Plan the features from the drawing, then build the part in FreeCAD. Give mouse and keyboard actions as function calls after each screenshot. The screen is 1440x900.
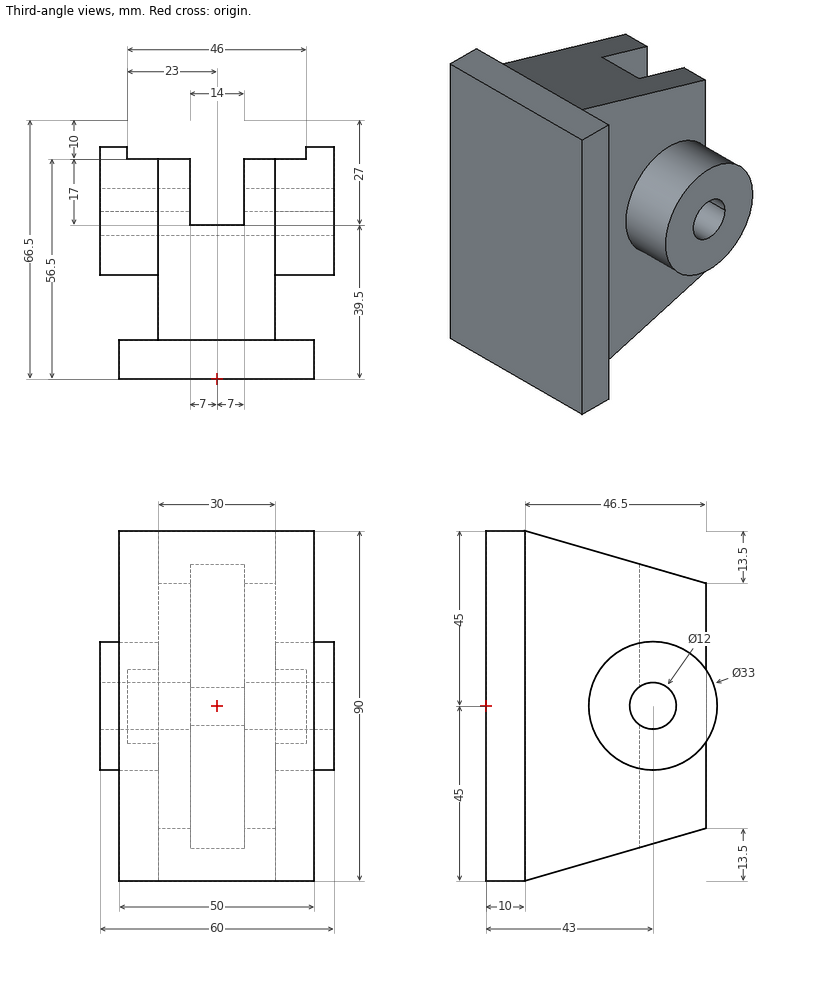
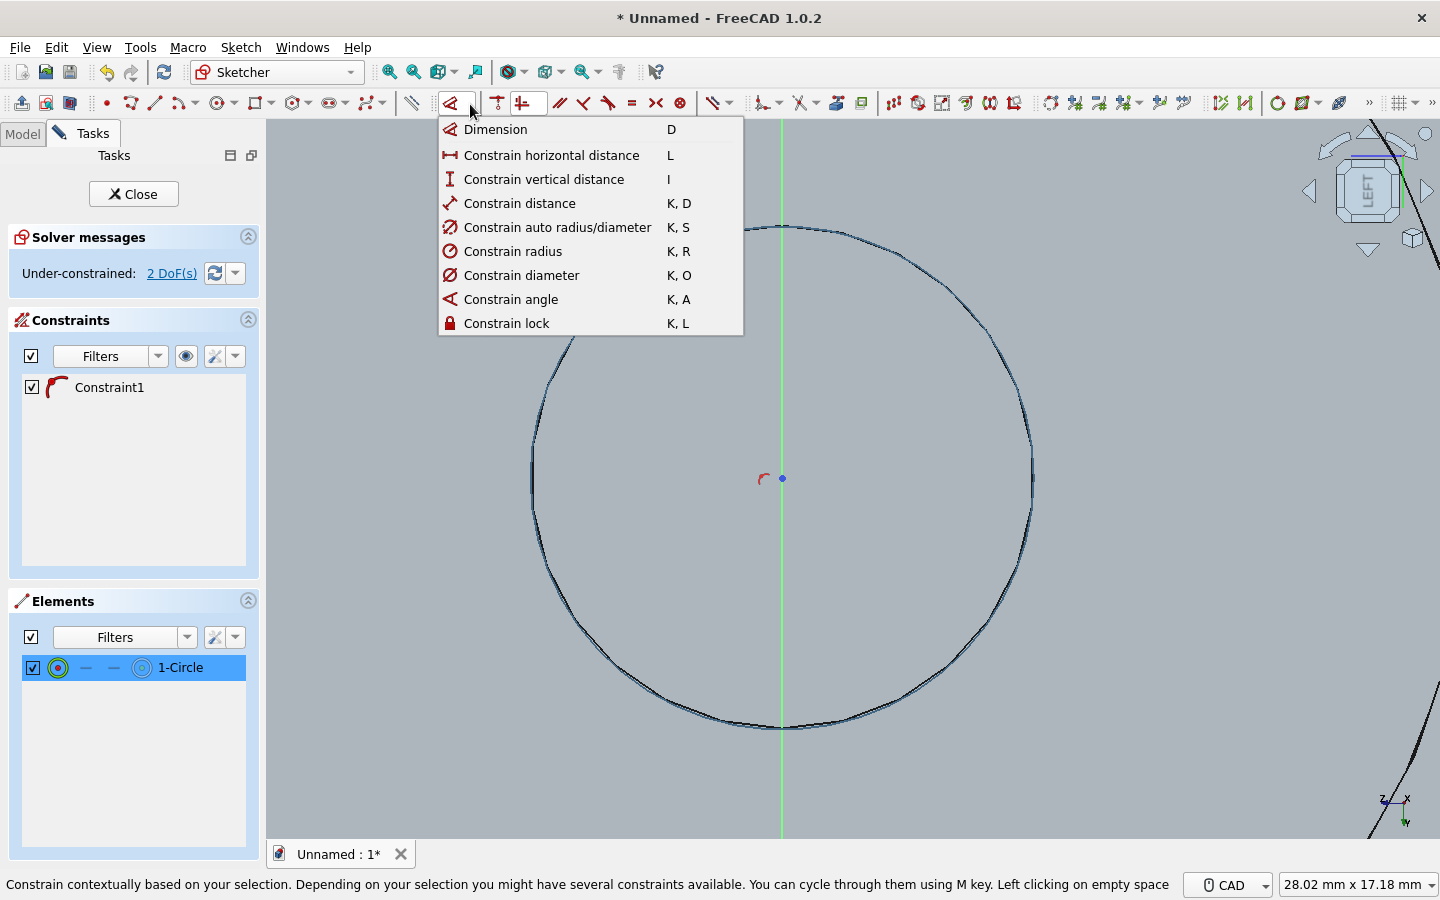
click(591, 275)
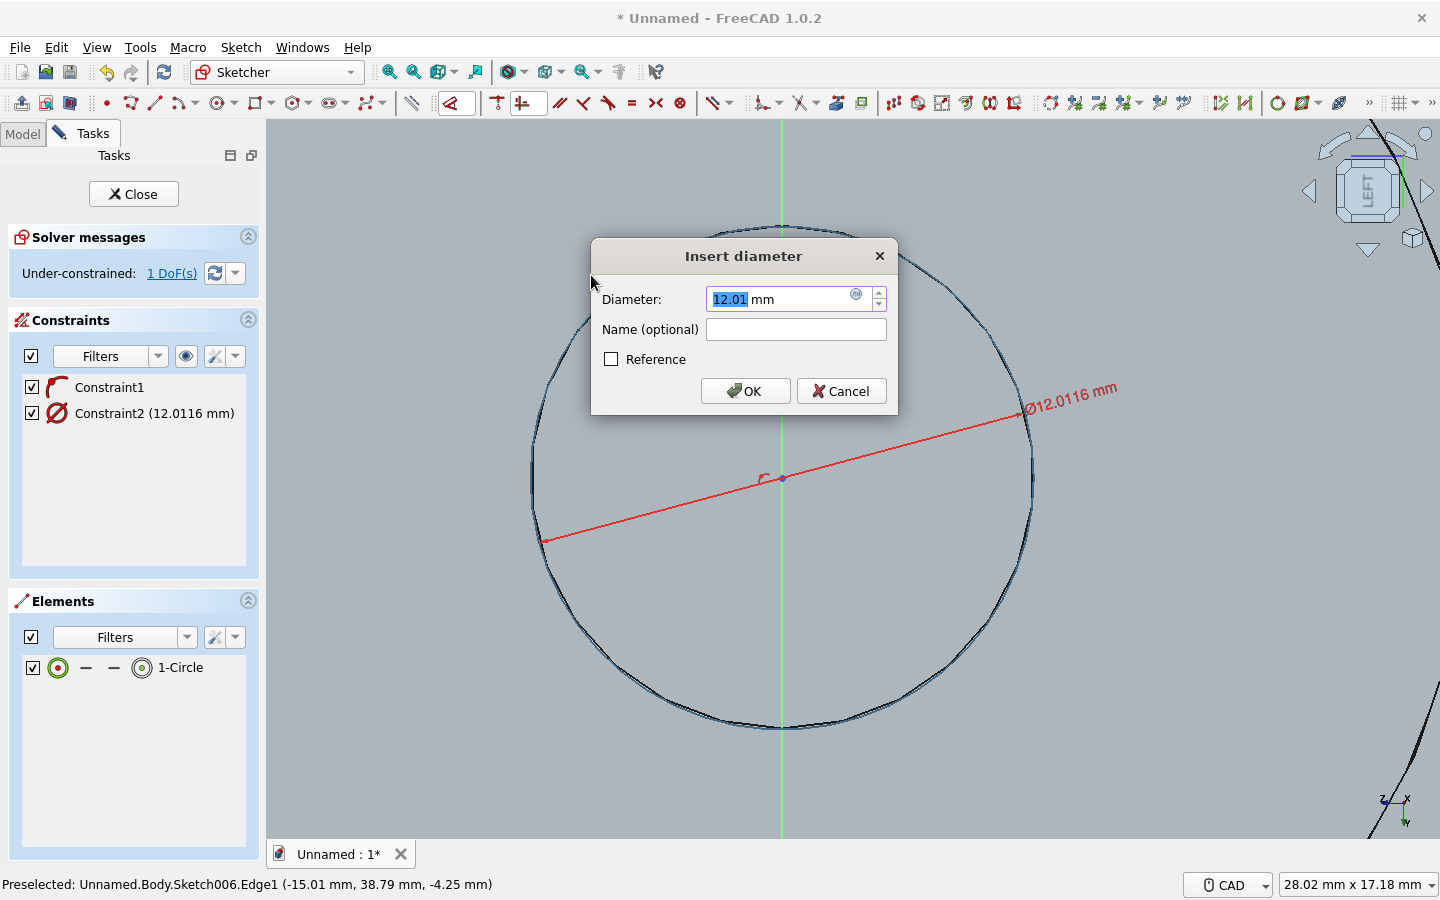
text(12)
key(Return)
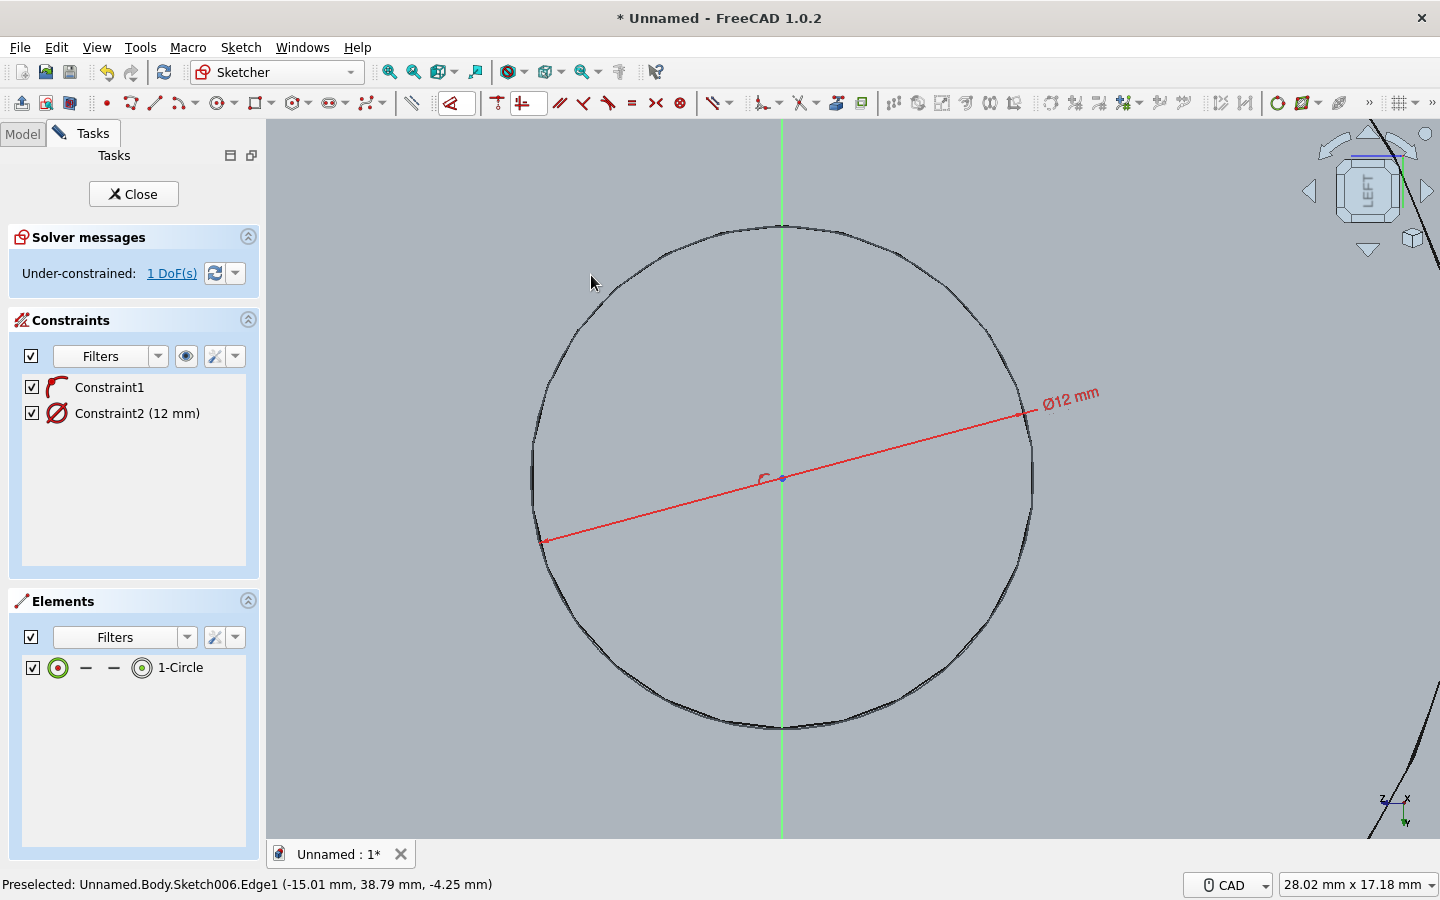
click(782, 478)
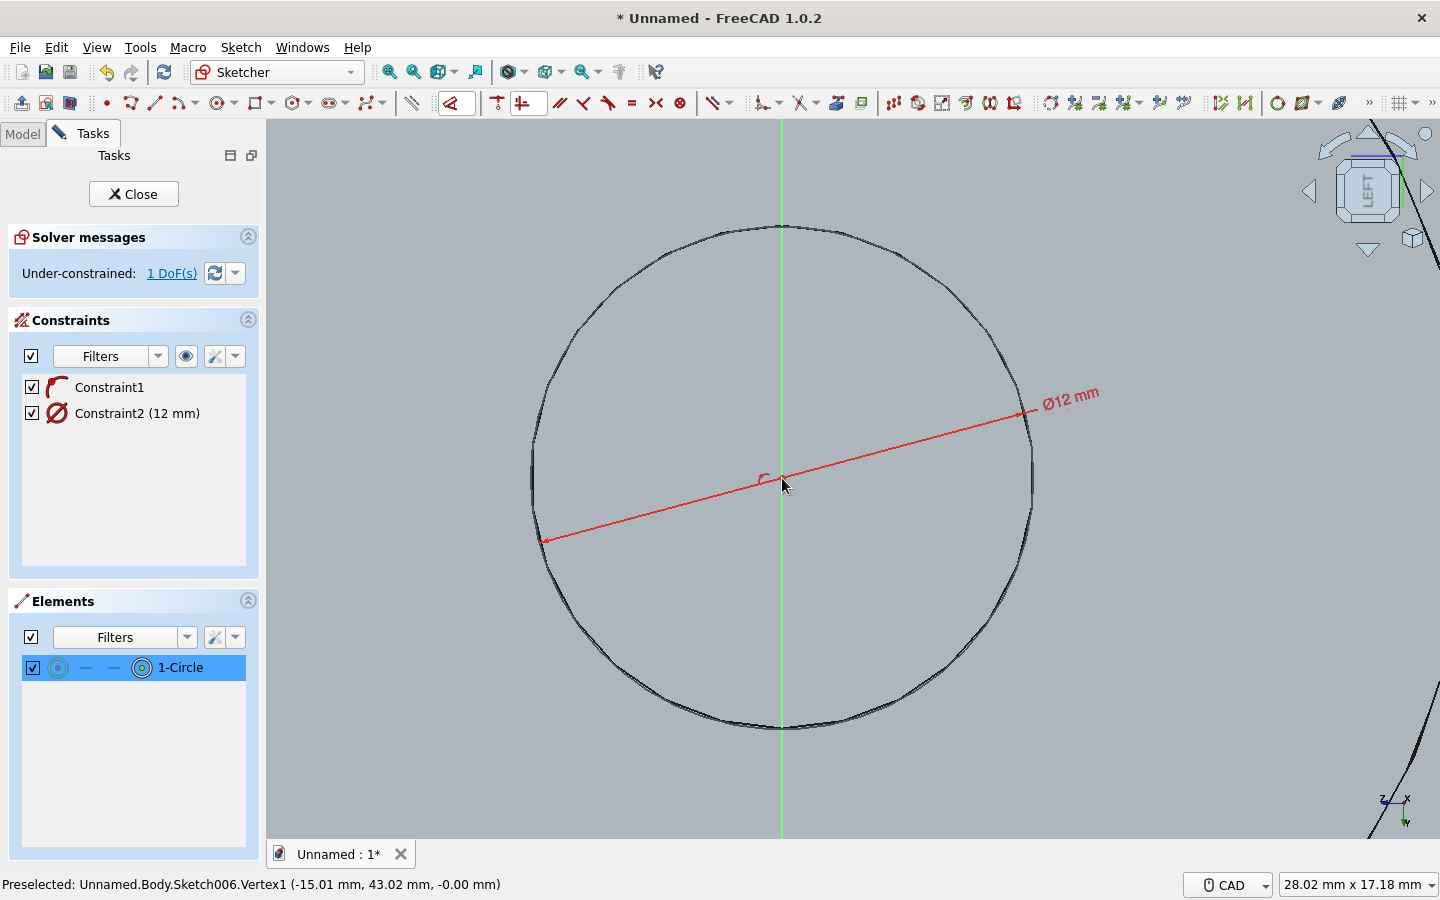
click(470, 104)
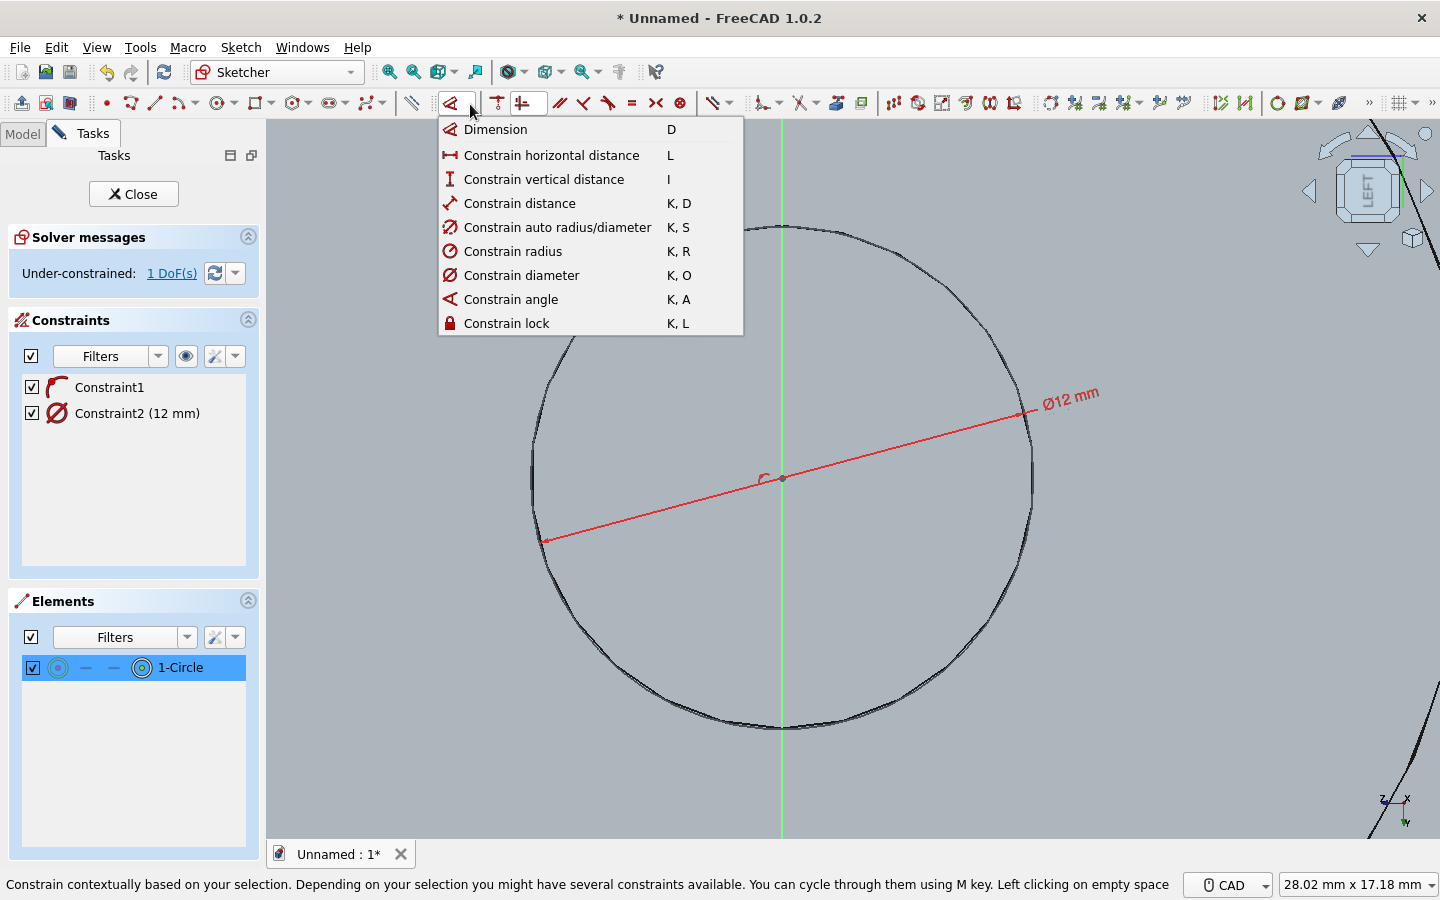
click(591, 179)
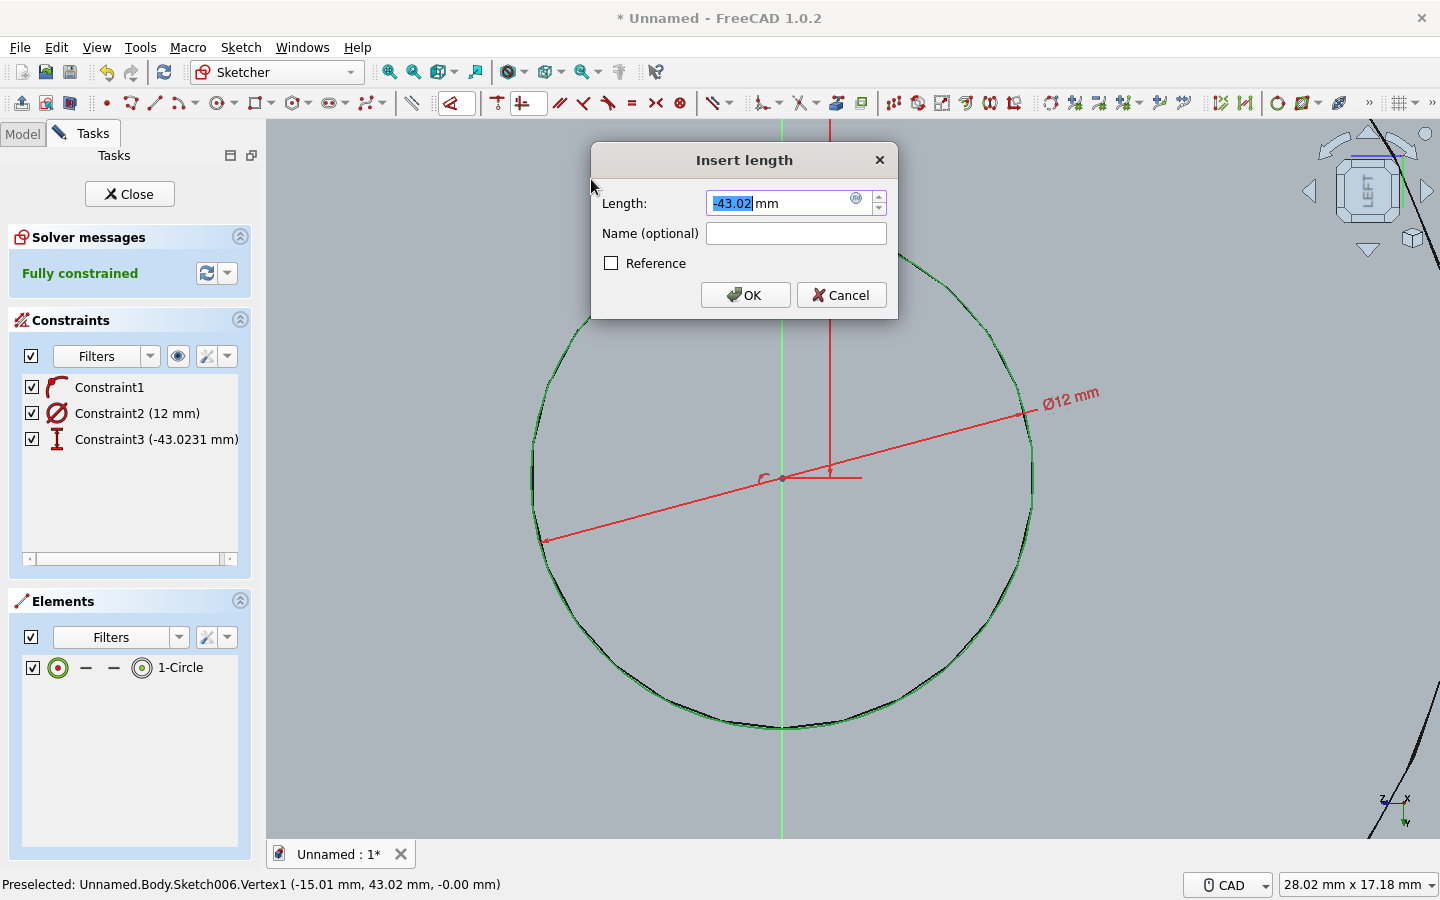
text(-43)
key(Return)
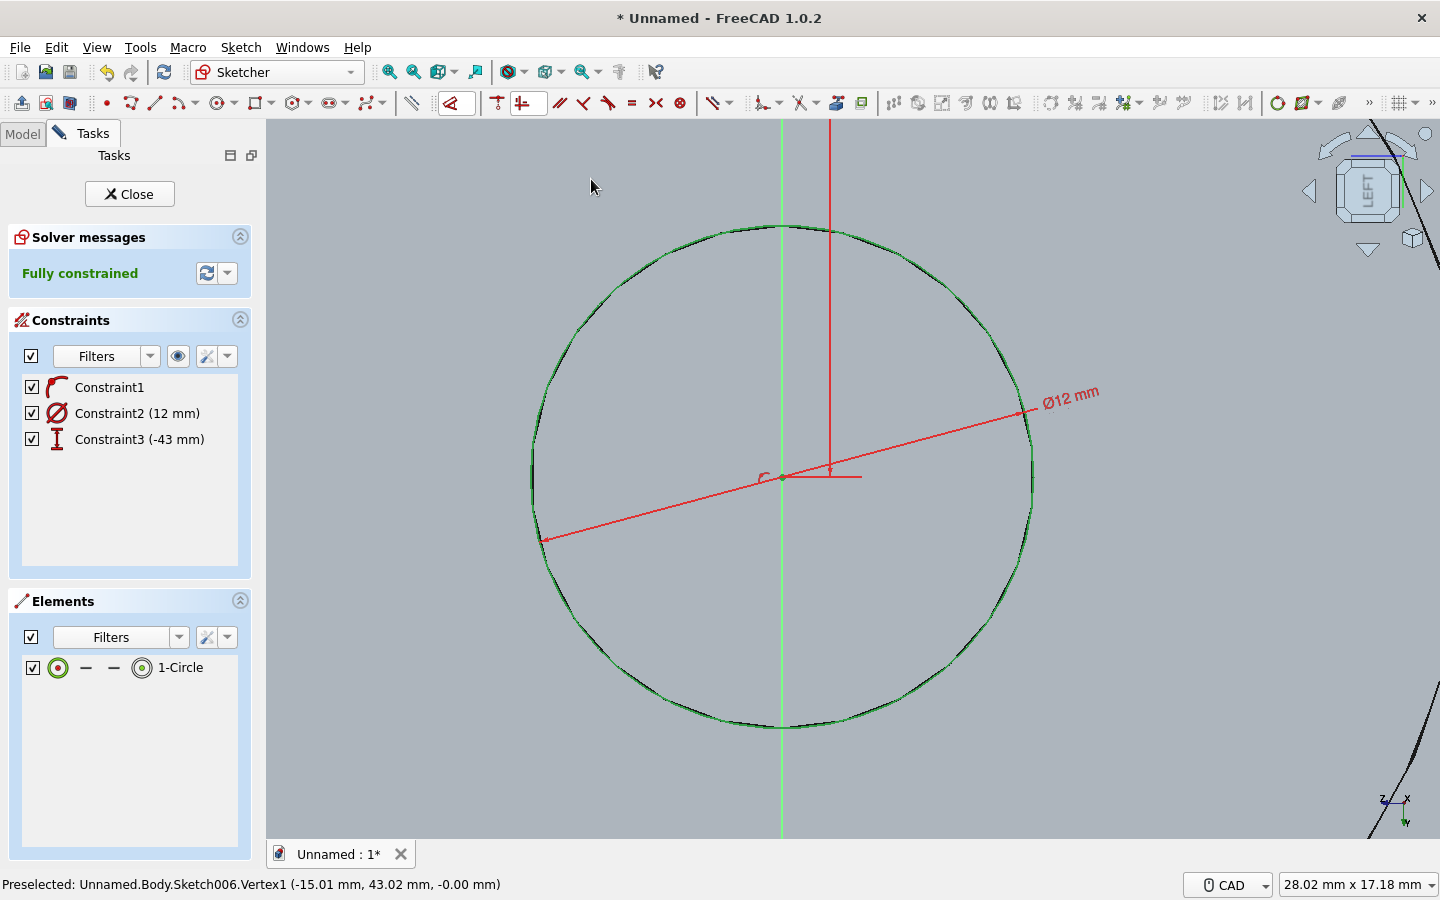
click(130, 194)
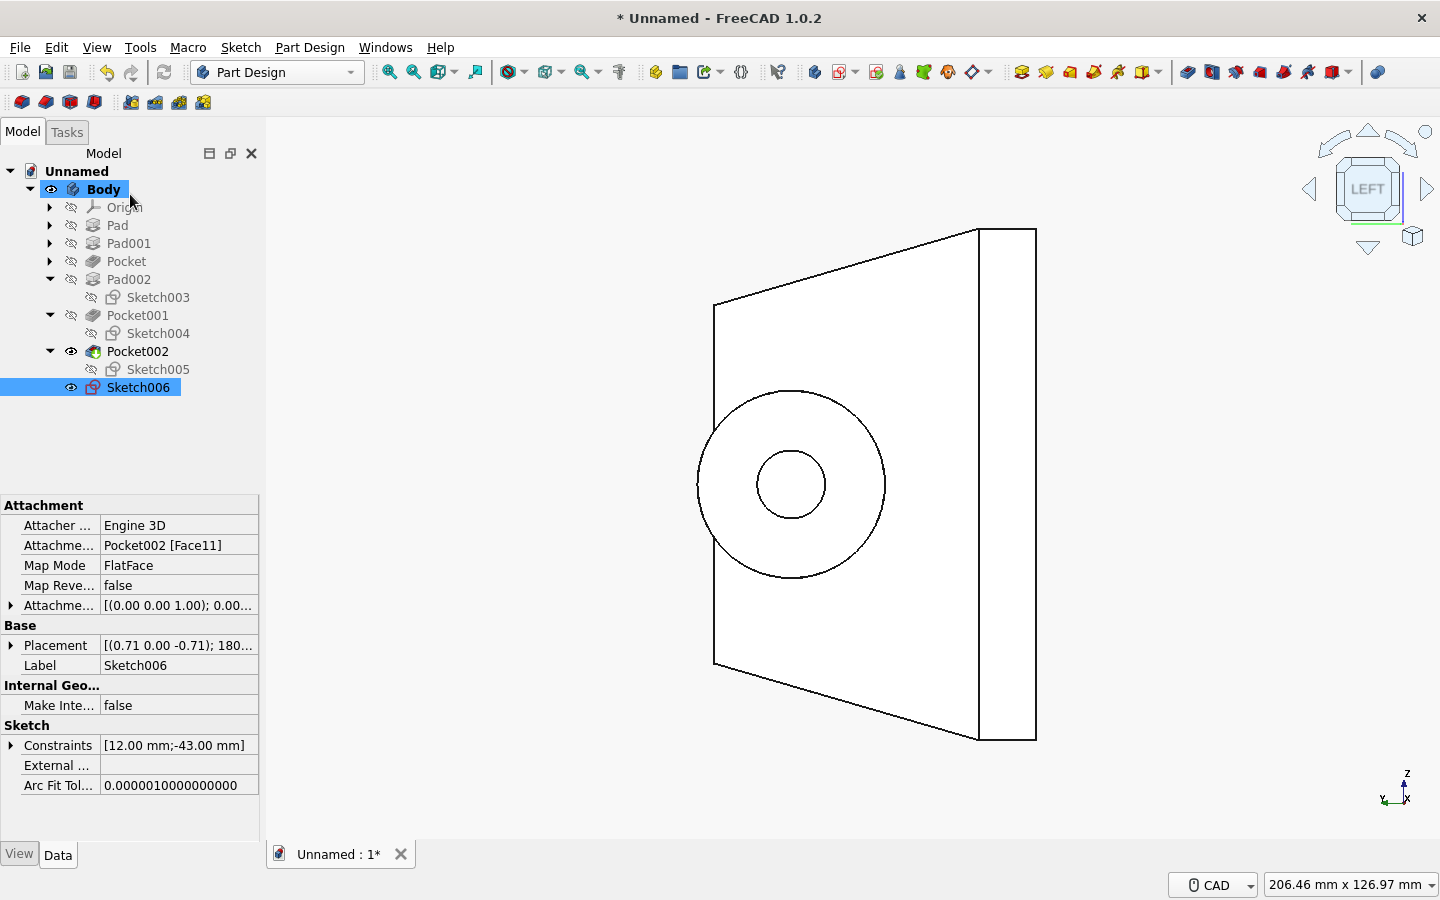
click(1188, 72)